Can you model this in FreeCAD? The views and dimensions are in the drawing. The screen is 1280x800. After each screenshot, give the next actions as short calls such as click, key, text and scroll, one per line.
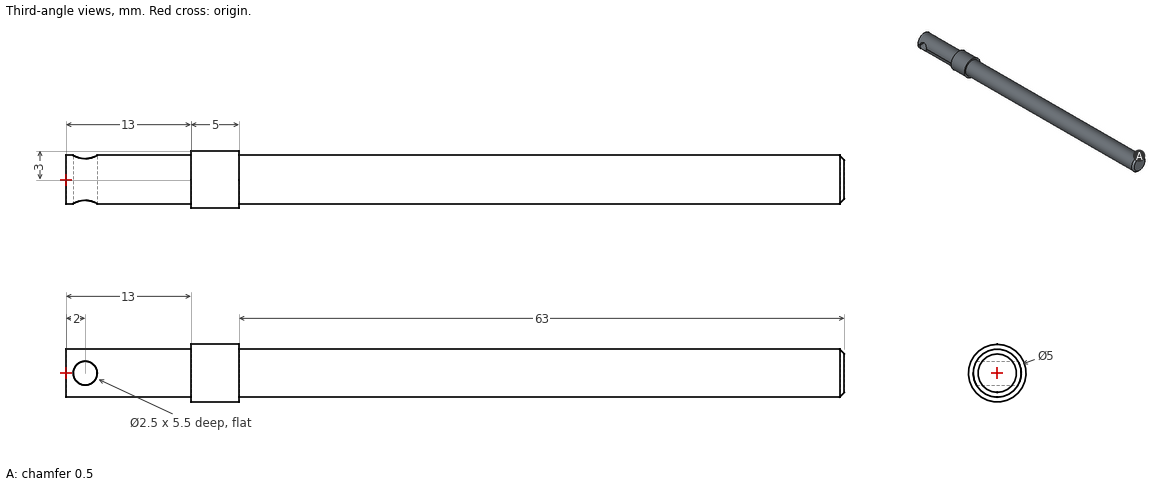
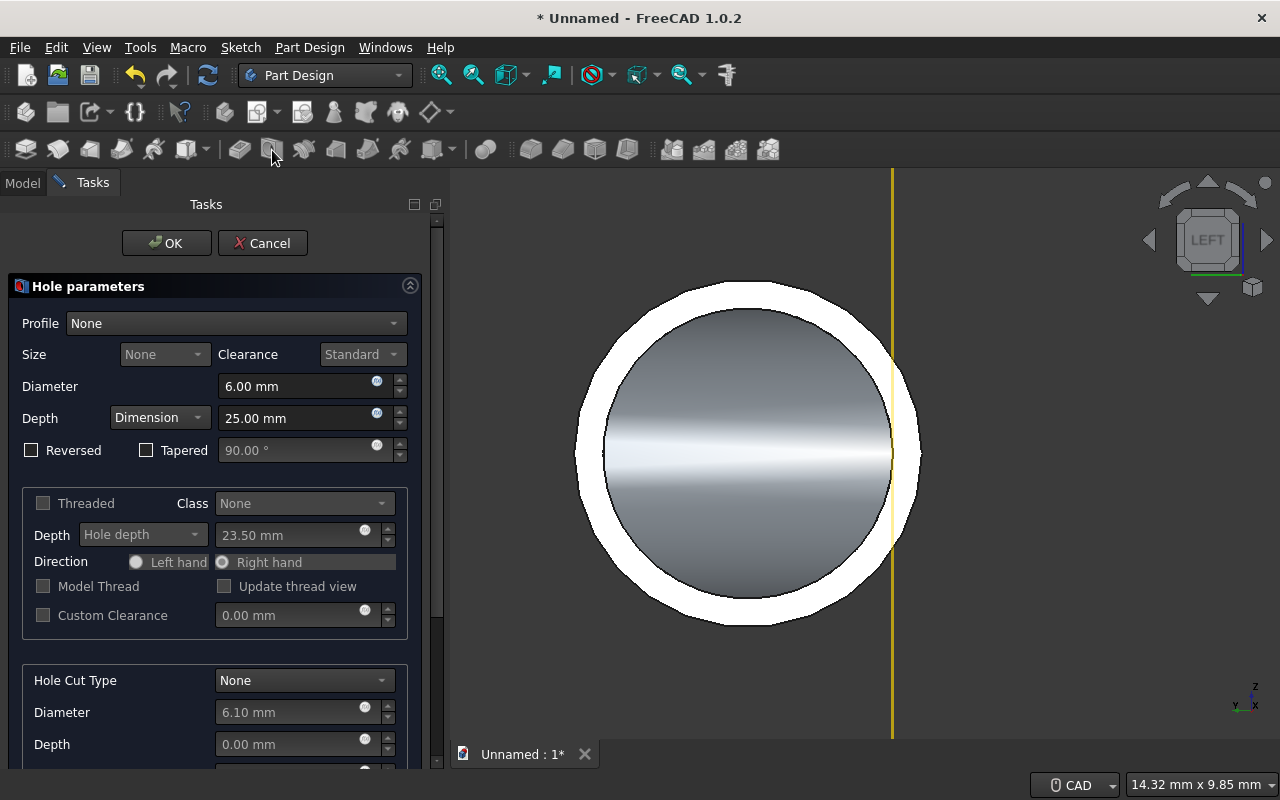
triple_click(305, 386)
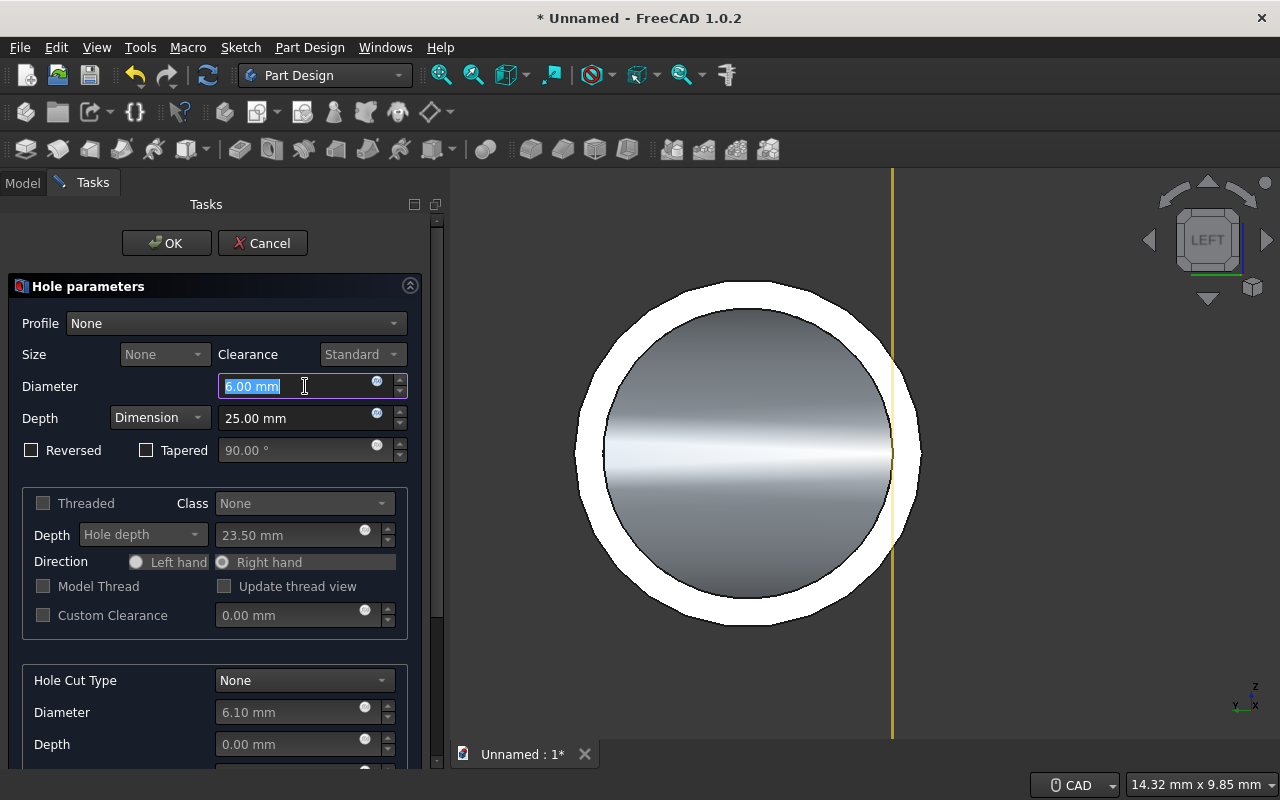
text(2.5)
key(Tab)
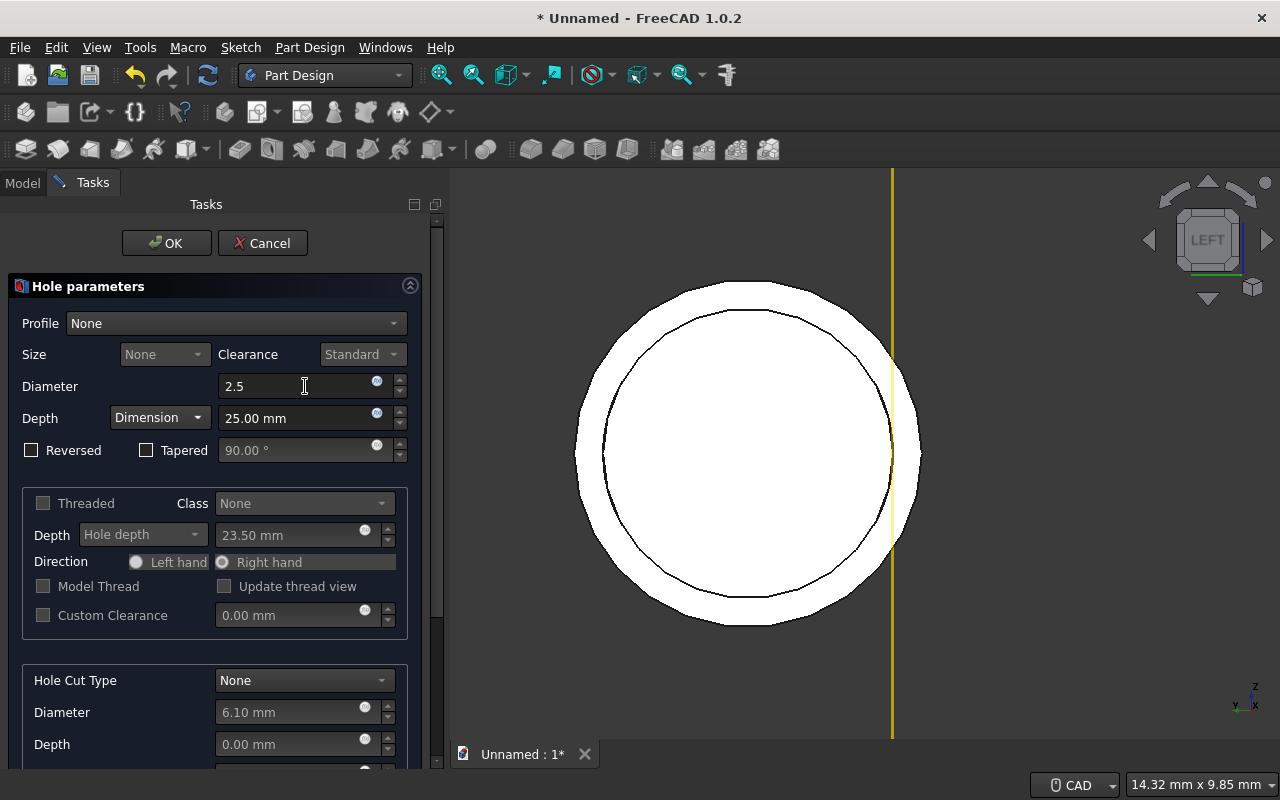
triple_click(305, 418)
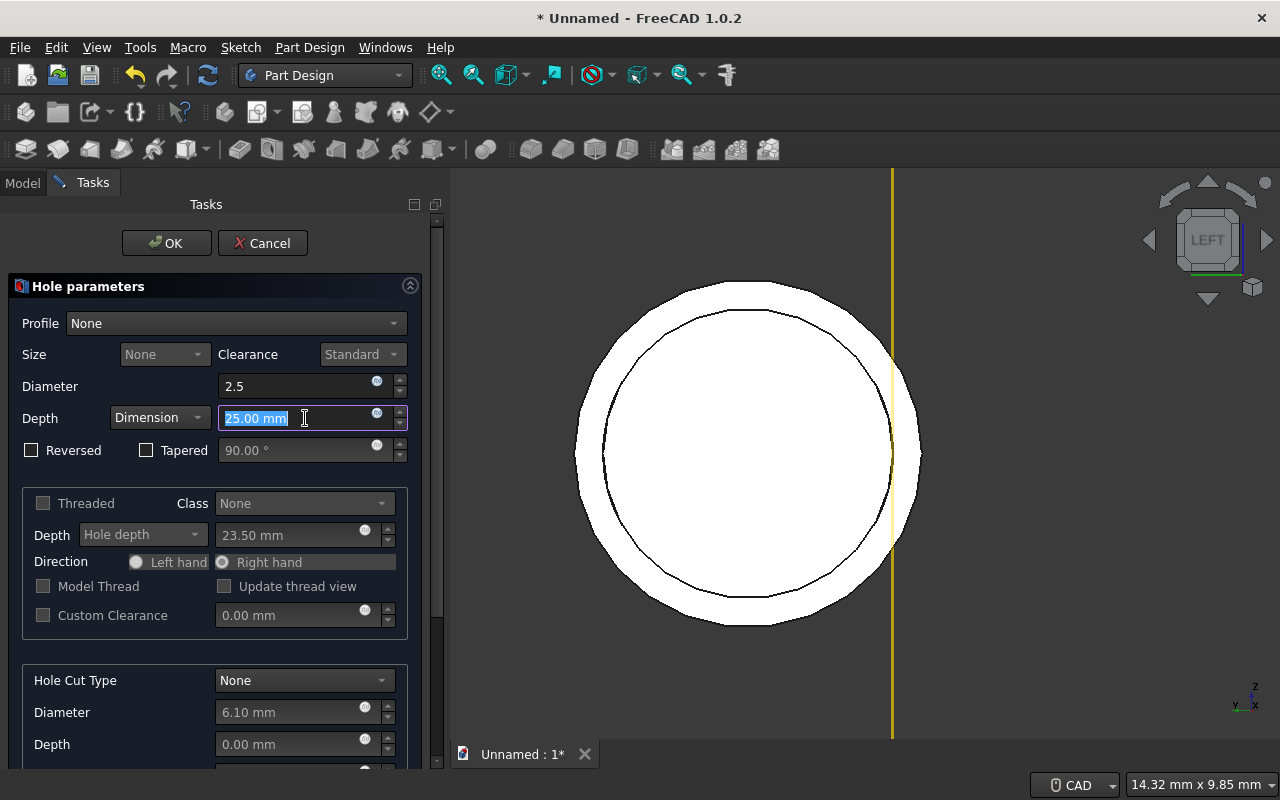
text(5.5)
key(Tab)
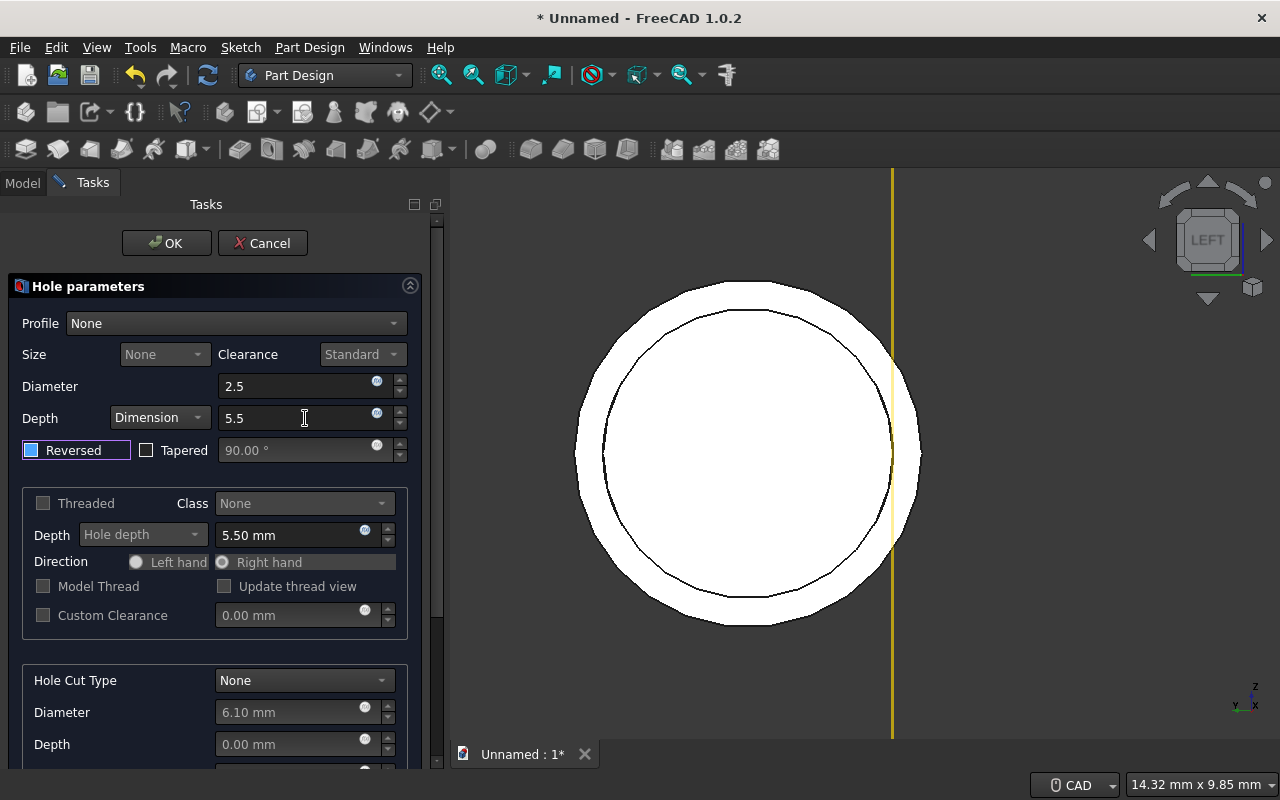
scroll(437, 491, down, 3)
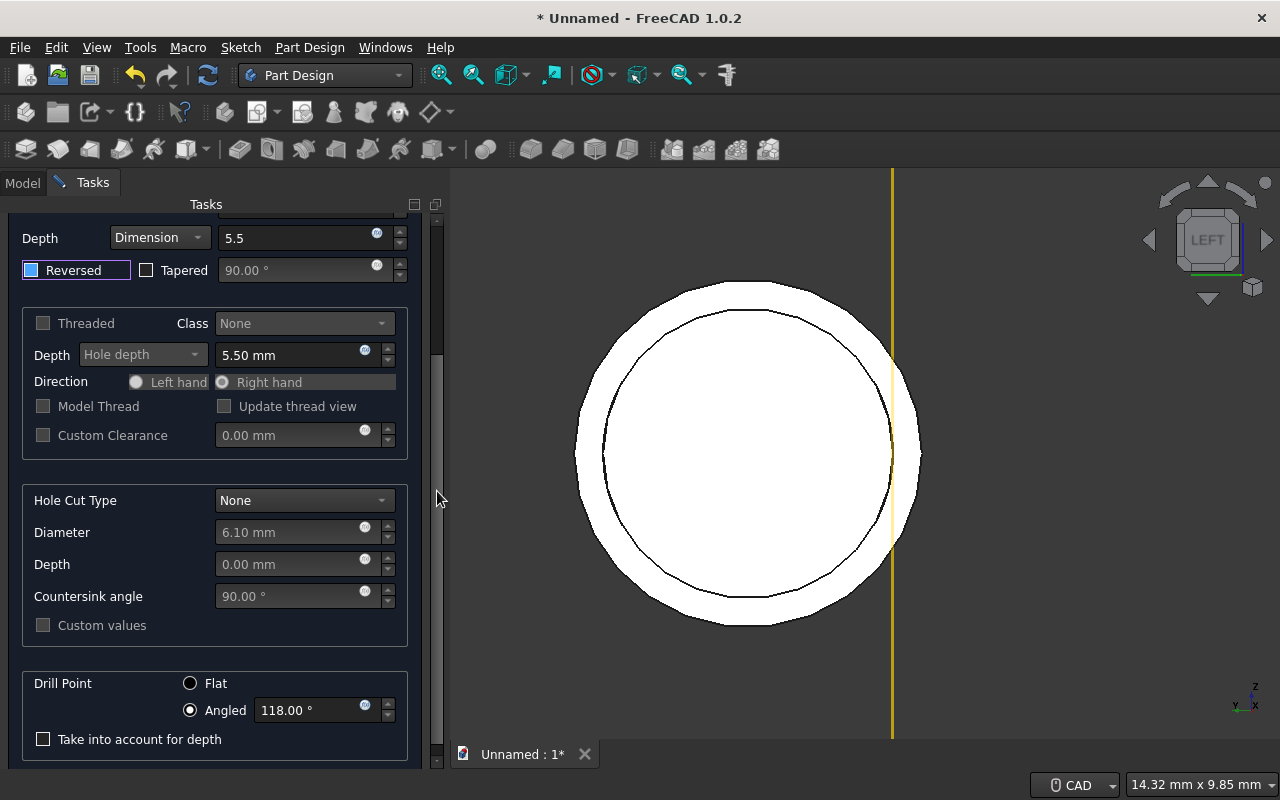
click(191, 683)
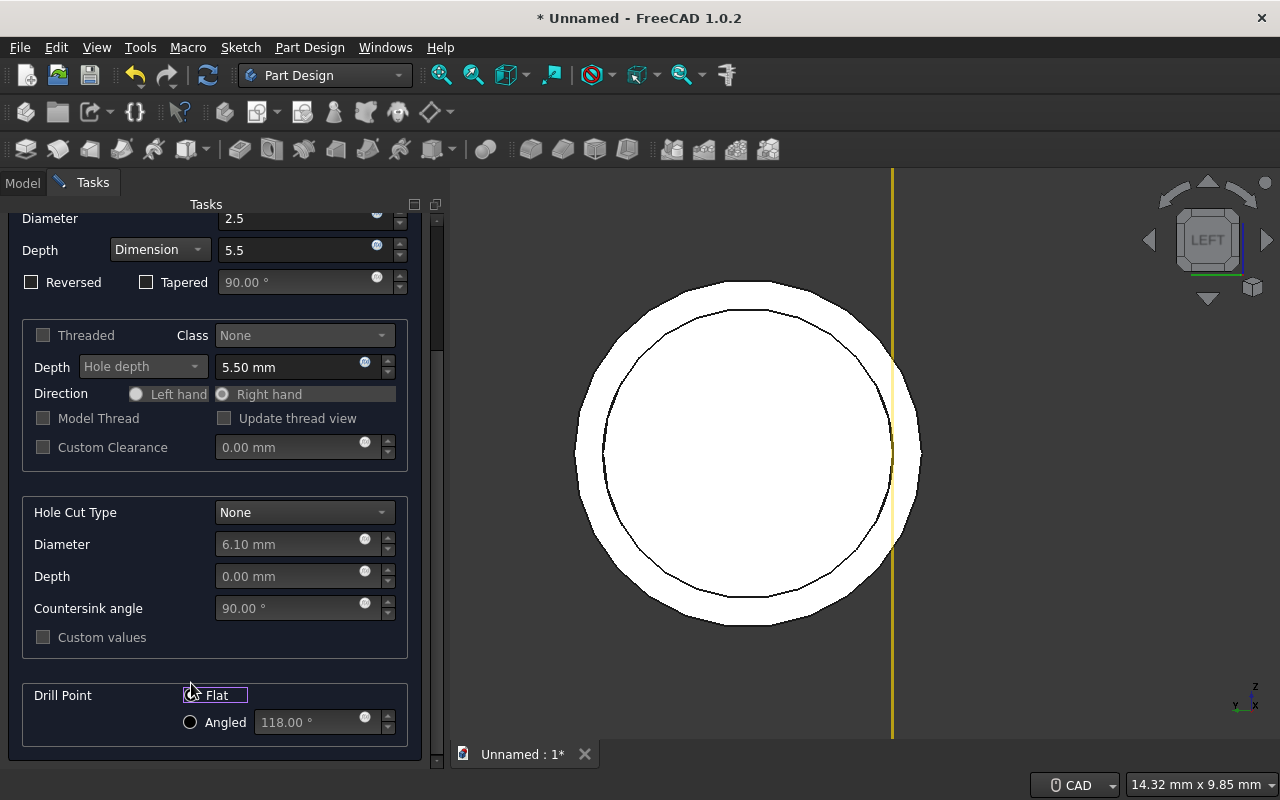
scroll(437, 491, up, 4)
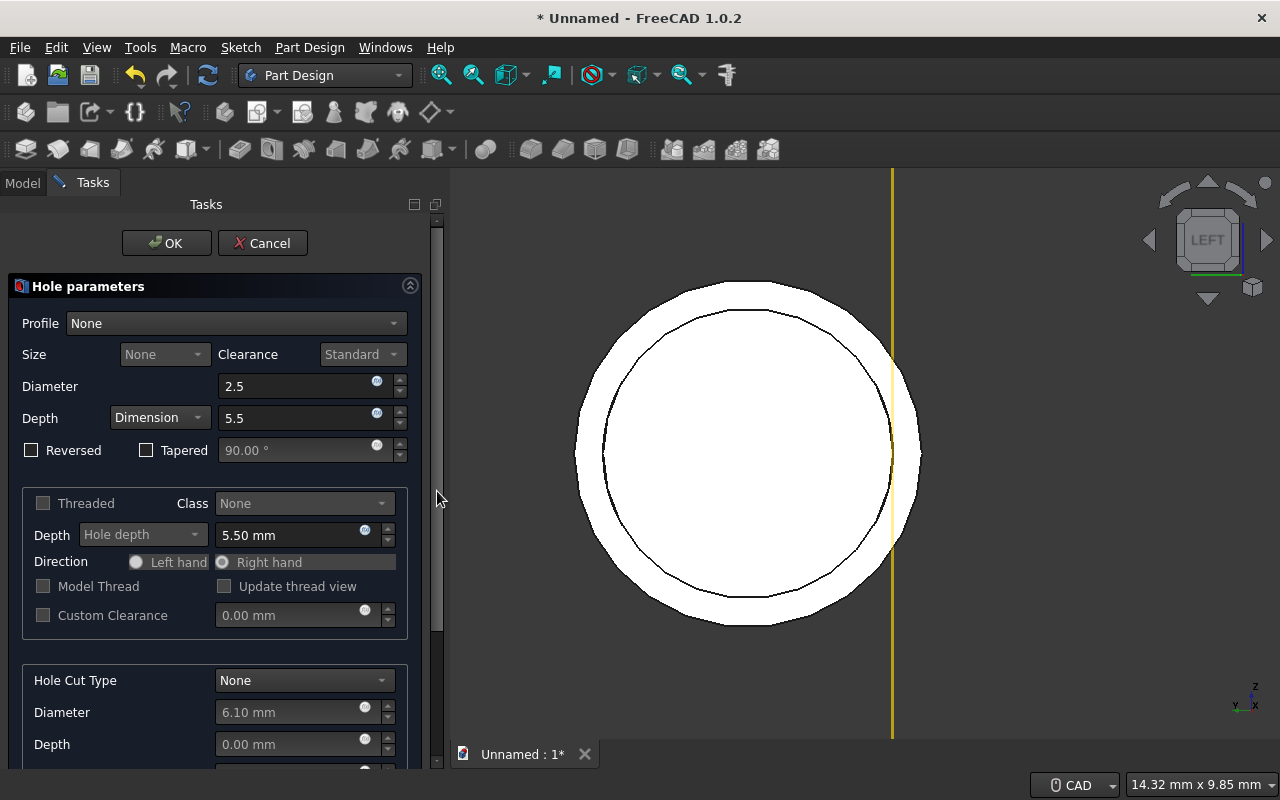
click(167, 243)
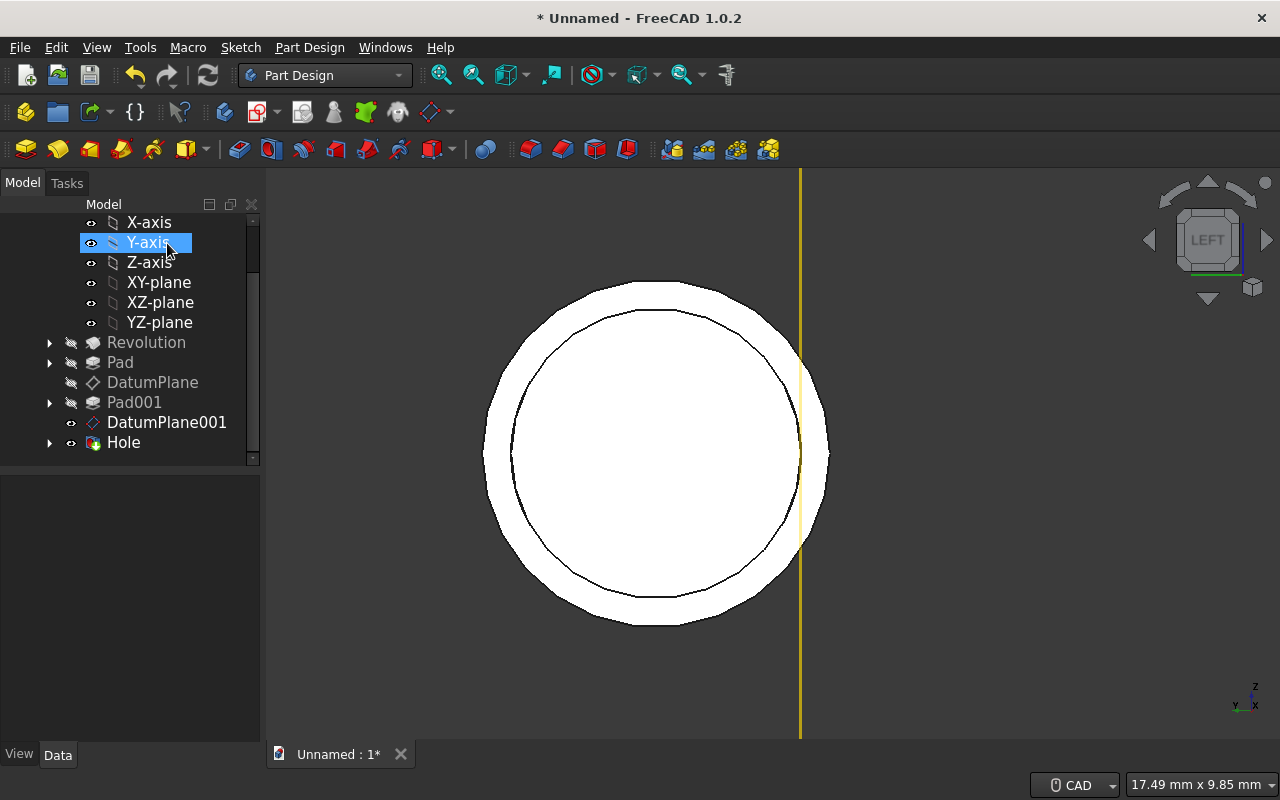
click(116, 423)
key(space)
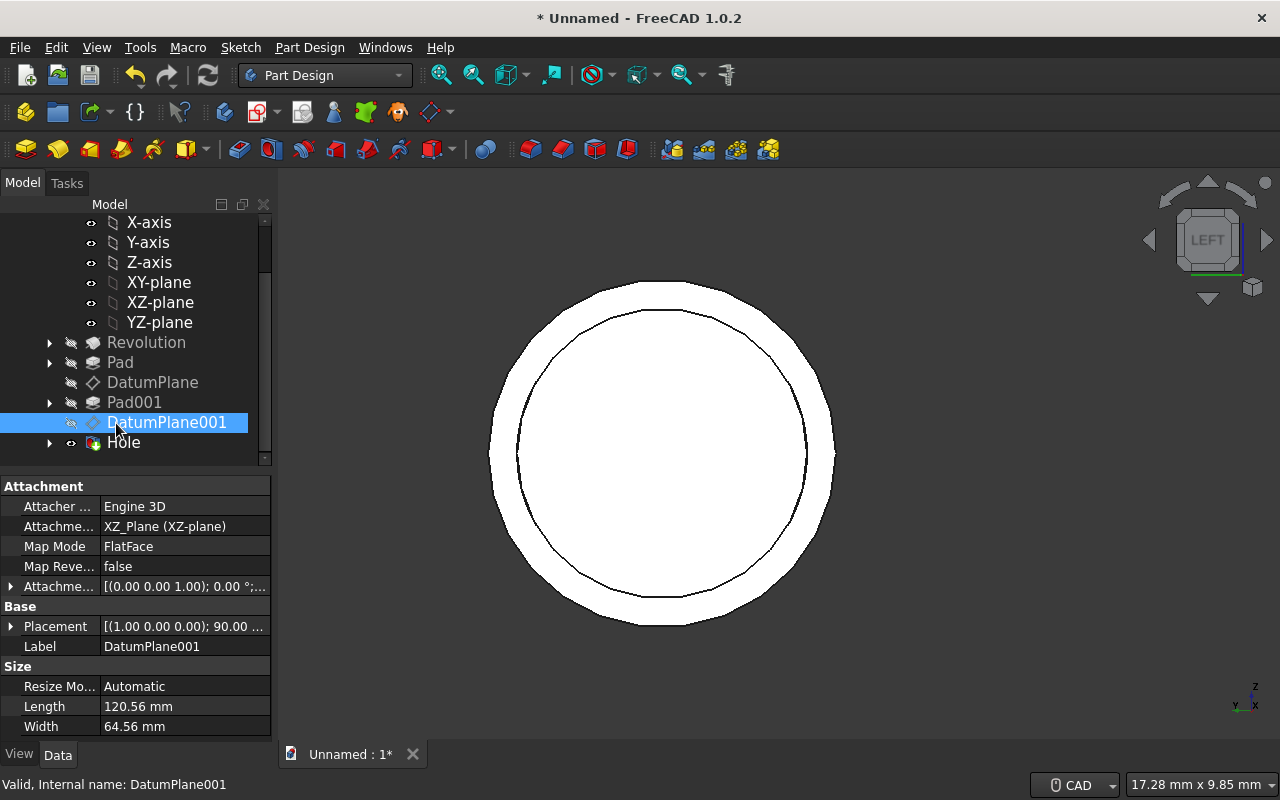
key(0)